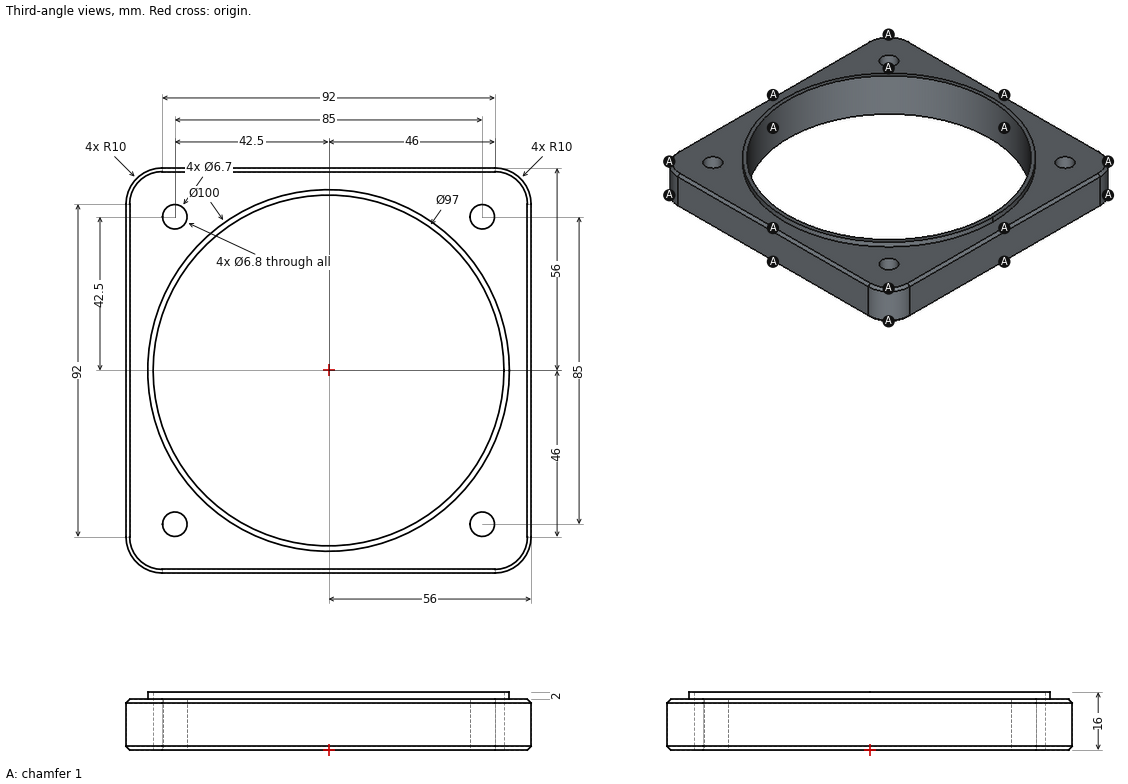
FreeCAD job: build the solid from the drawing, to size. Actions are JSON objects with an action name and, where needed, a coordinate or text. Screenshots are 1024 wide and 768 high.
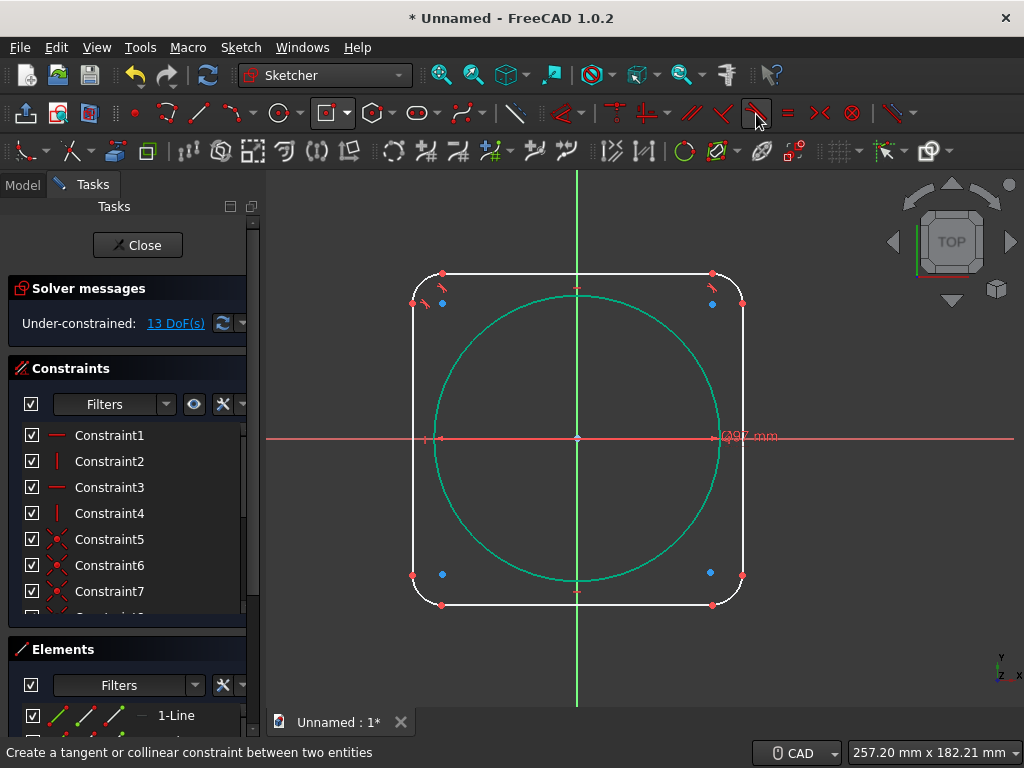
{"action": "left_click", "coordinate": [413, 385]}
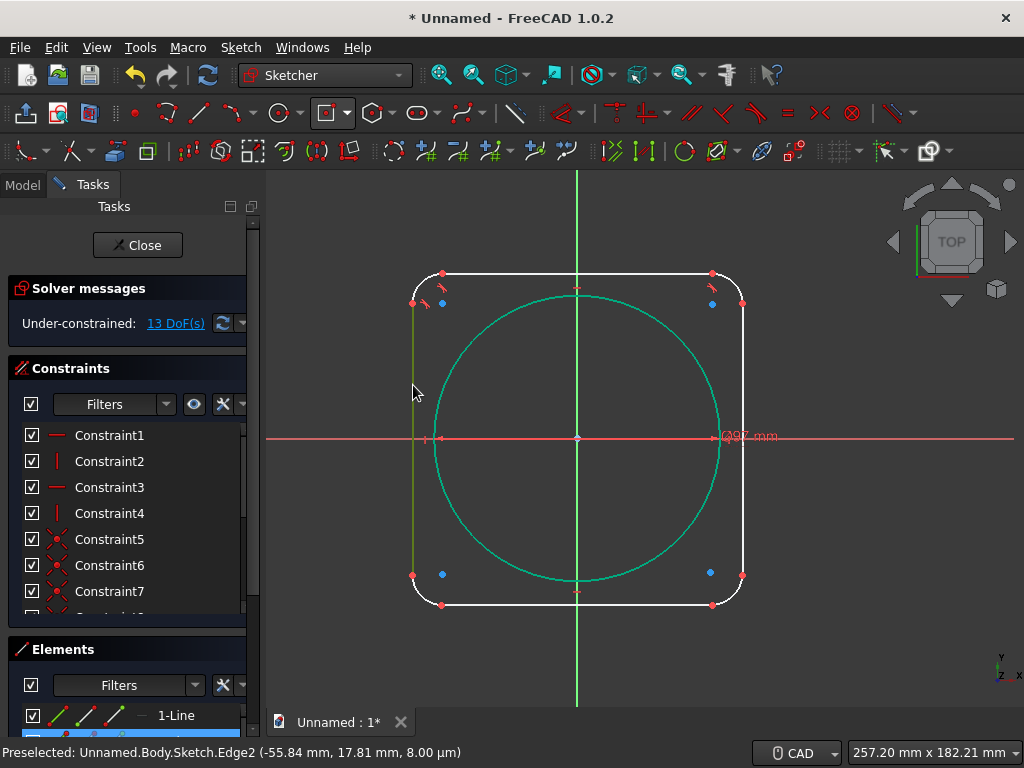
{"action": "left_click", "coordinate": [416, 588]}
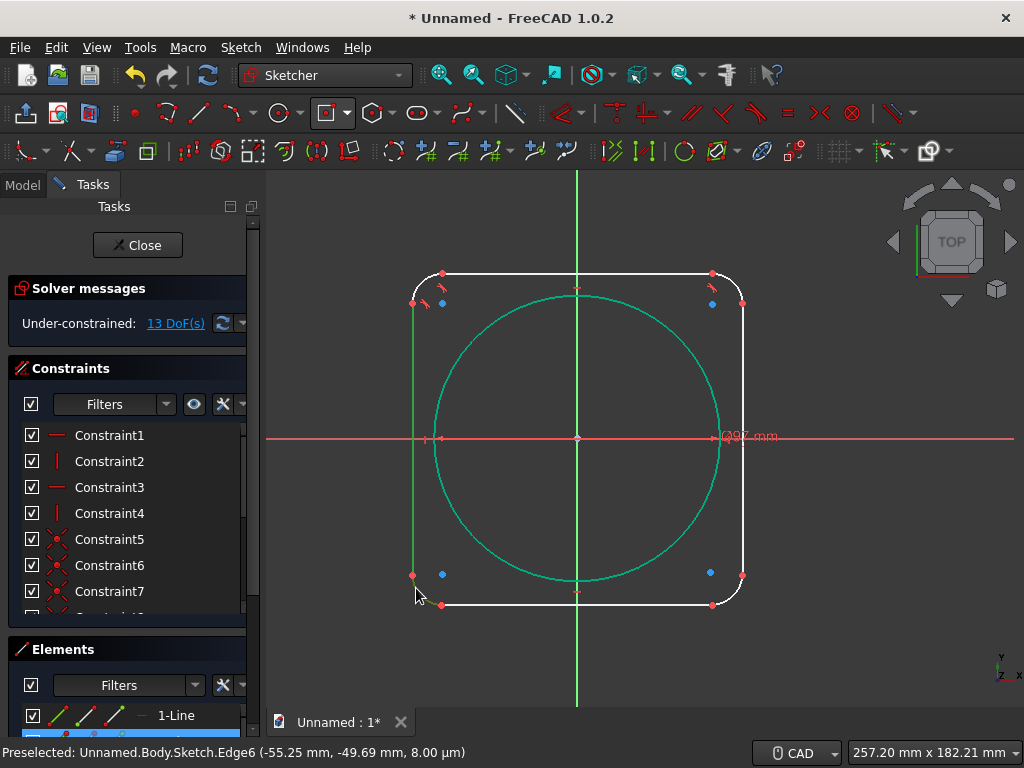
{"action": "left_click", "coordinate": [756, 114]}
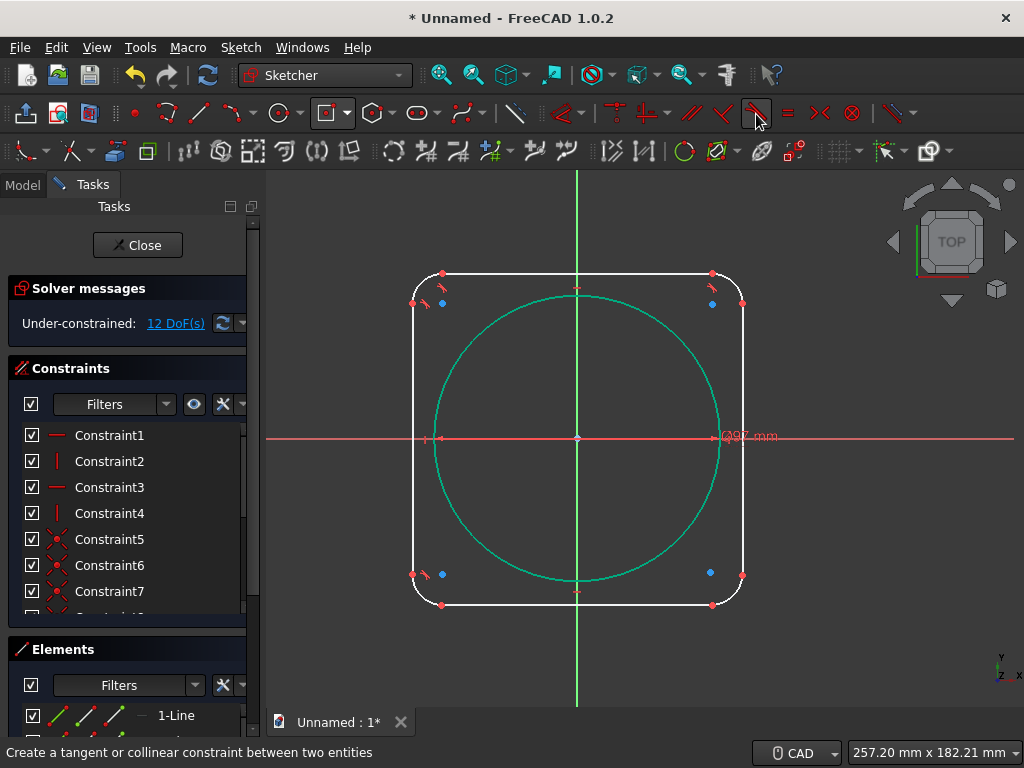
{"action": "left_click", "coordinate": [523, 605]}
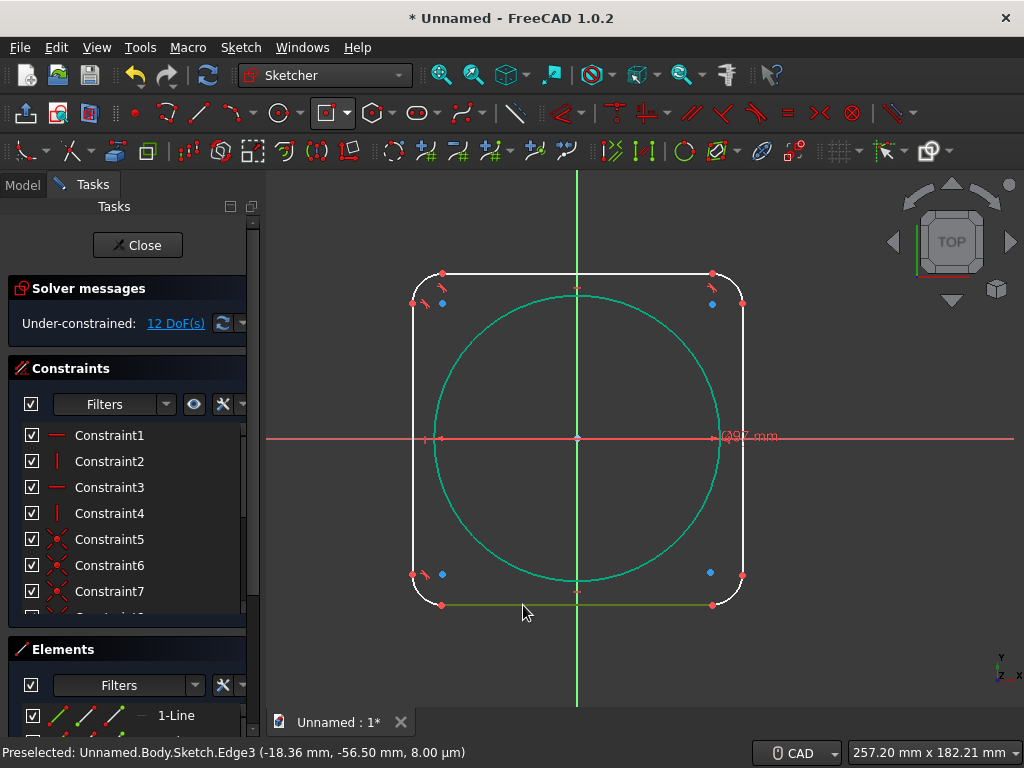
{"action": "left_click", "coordinate": [416, 588]}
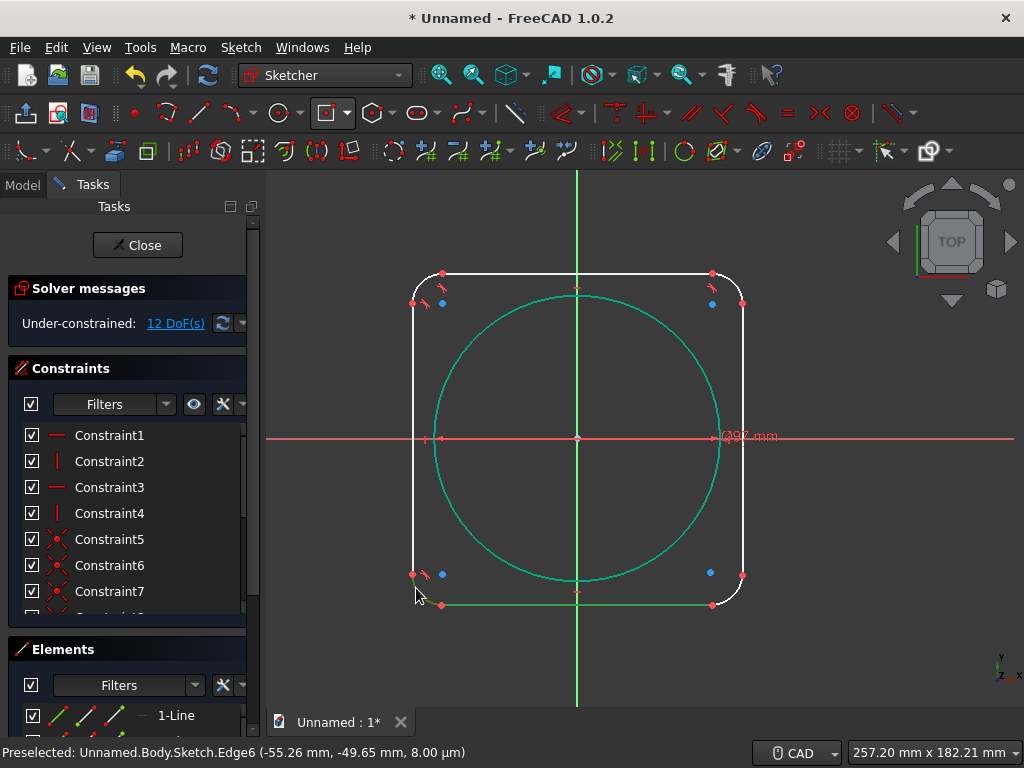
{"action": "left_click", "coordinate": [756, 114]}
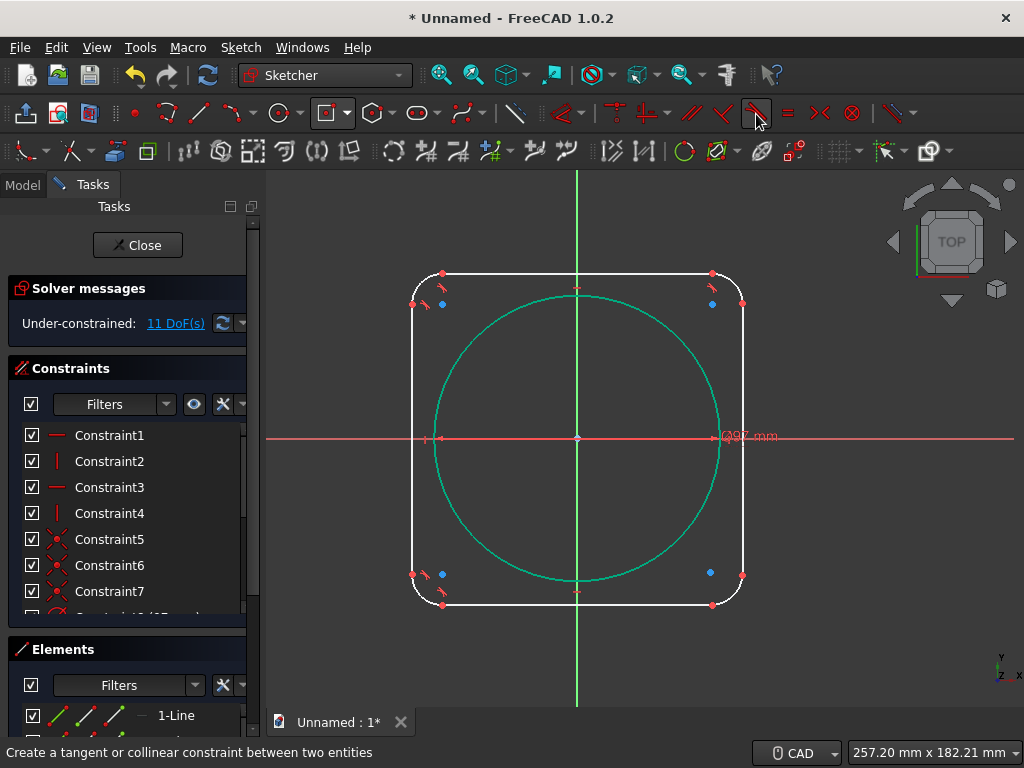
{"action": "left_click", "coordinate": [523, 605]}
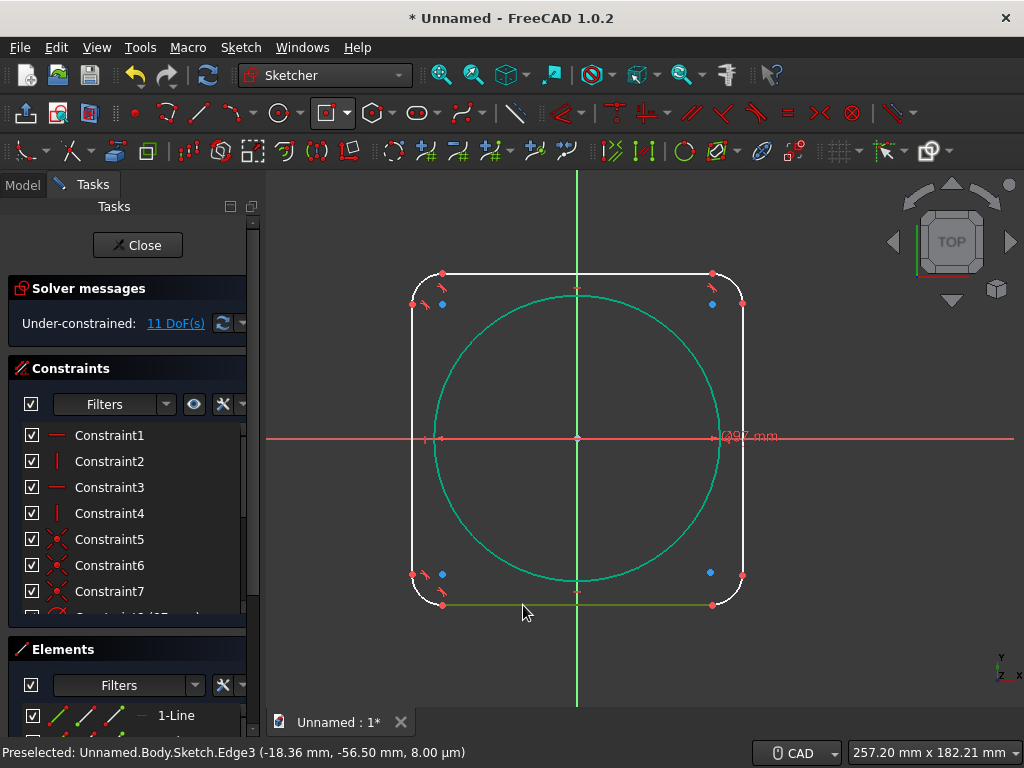
{"action": "left_click", "coordinate": [726, 601]}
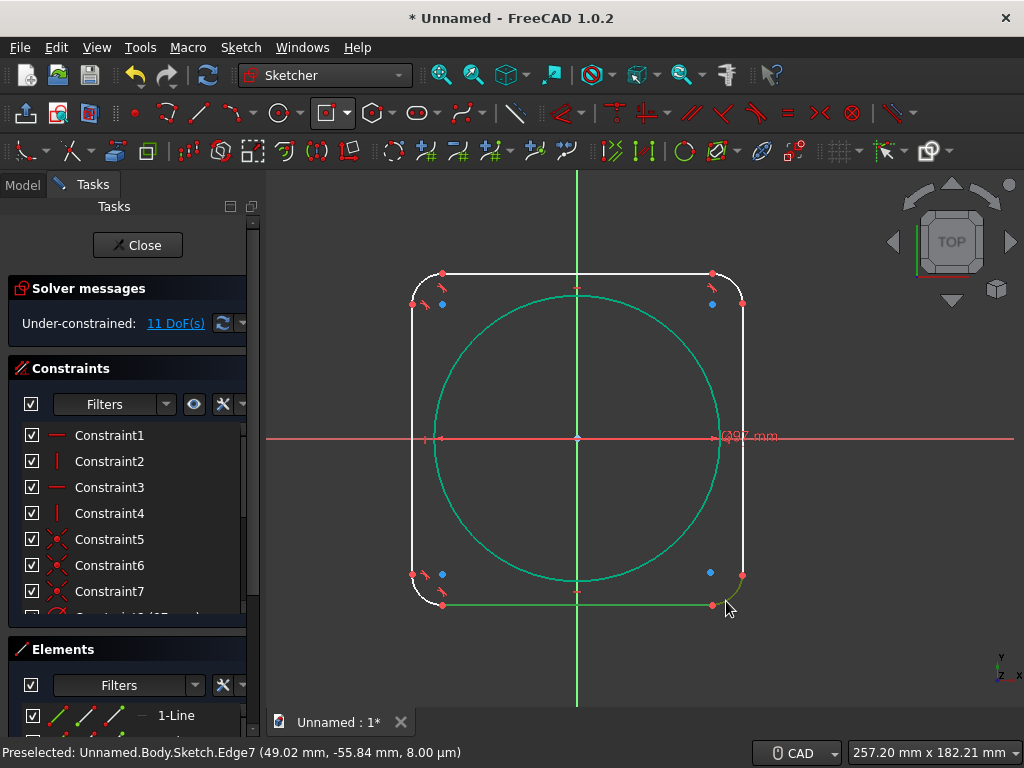
{"action": "left_click", "coordinate": [756, 114]}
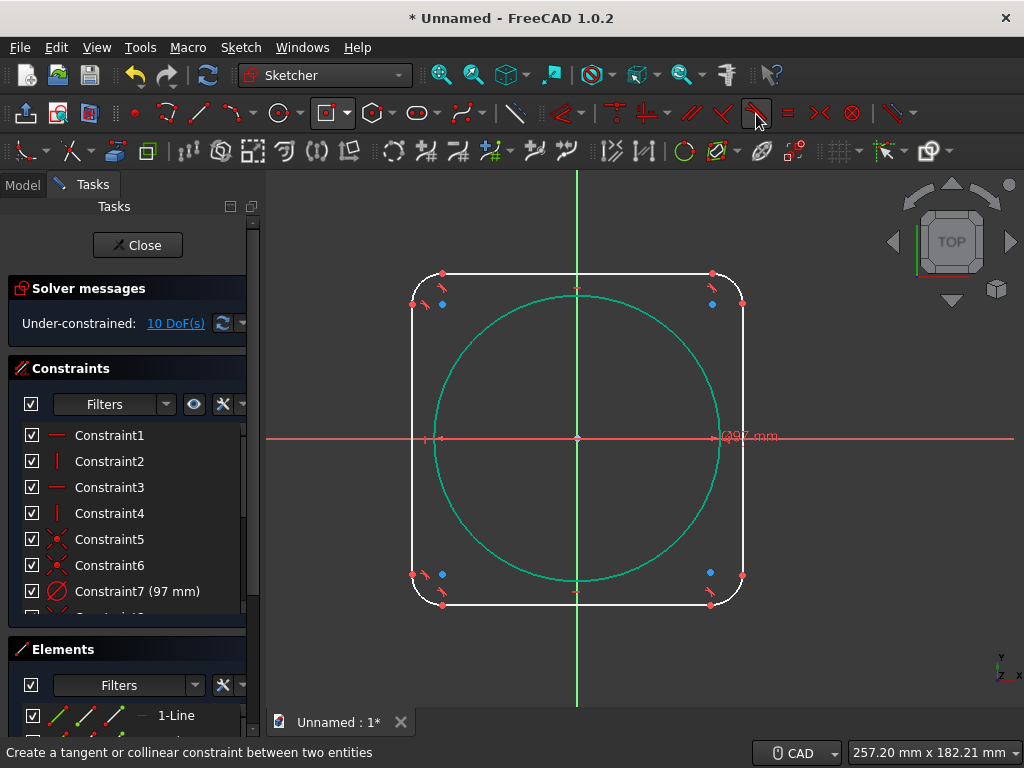
{"action": "left_click", "coordinate": [743, 494]}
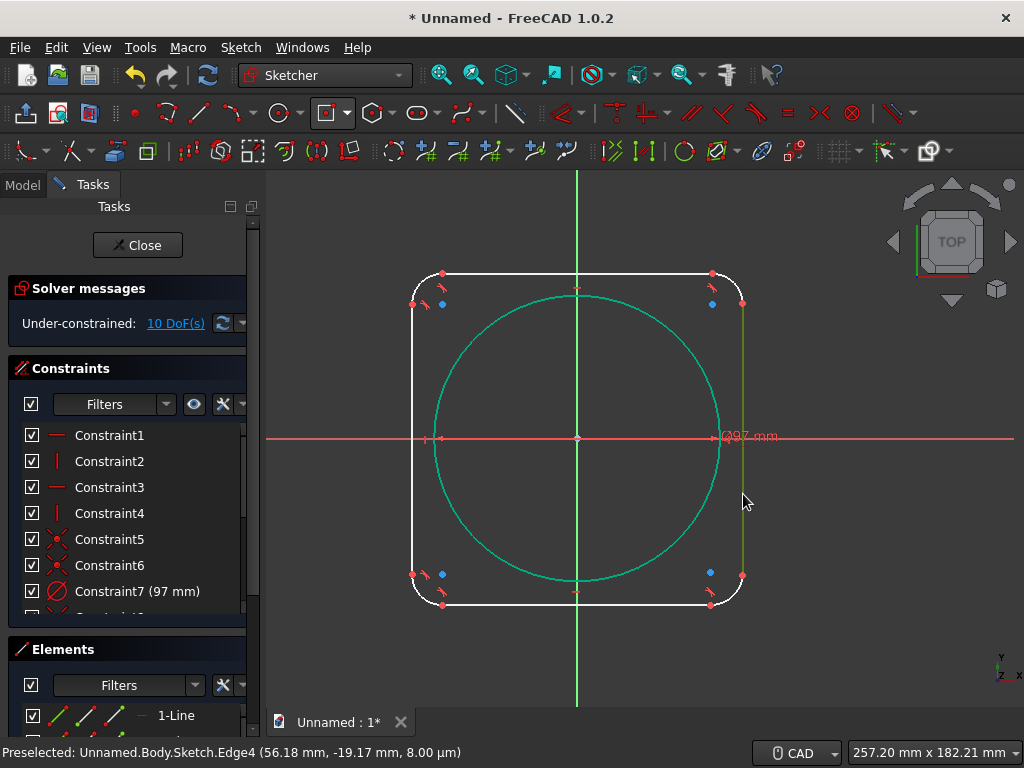
{"action": "left_click", "coordinate": [725, 602]}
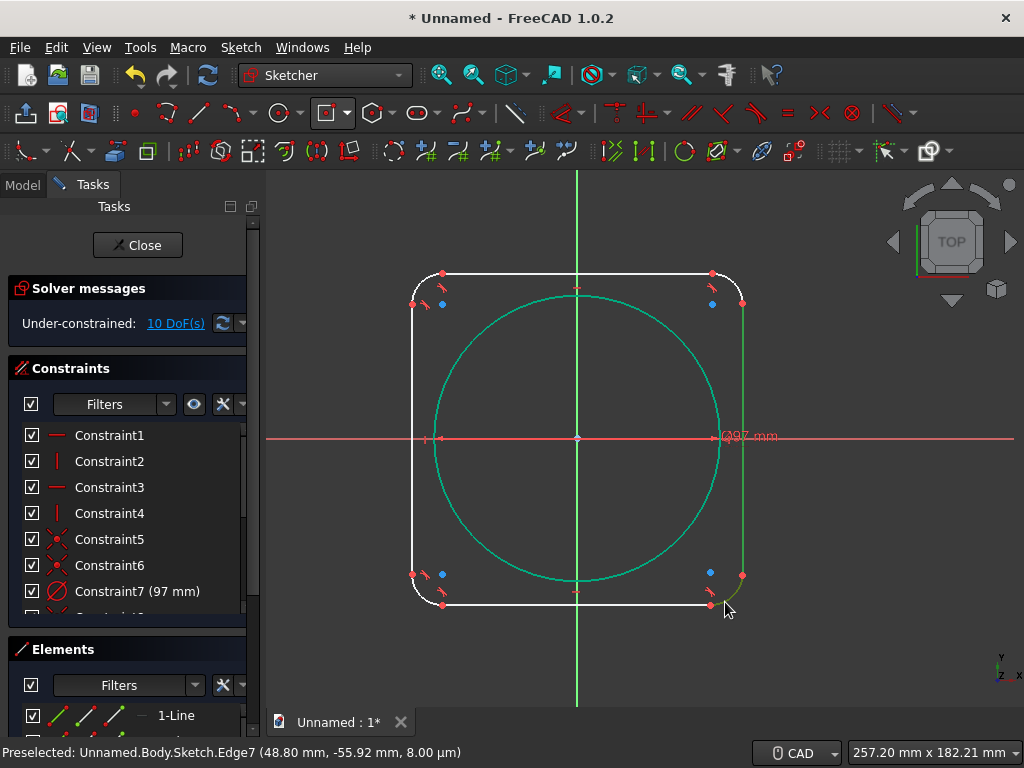
{"action": "left_click", "coordinate": [756, 114]}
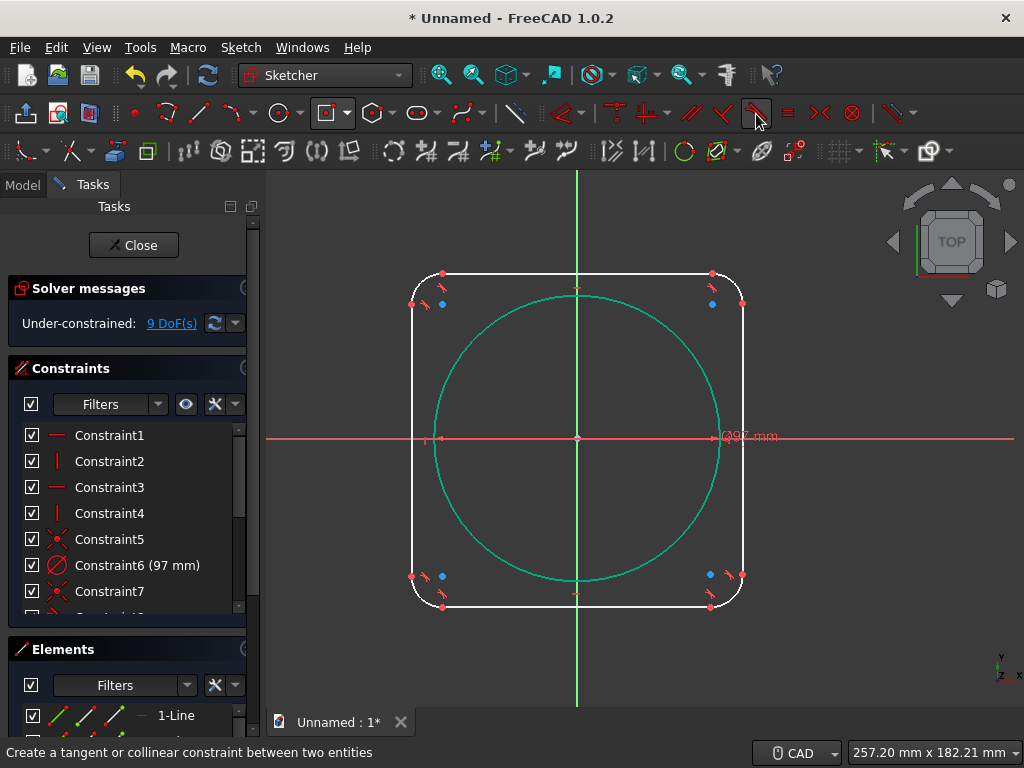
{"action": "left_click", "coordinate": [743, 494]}